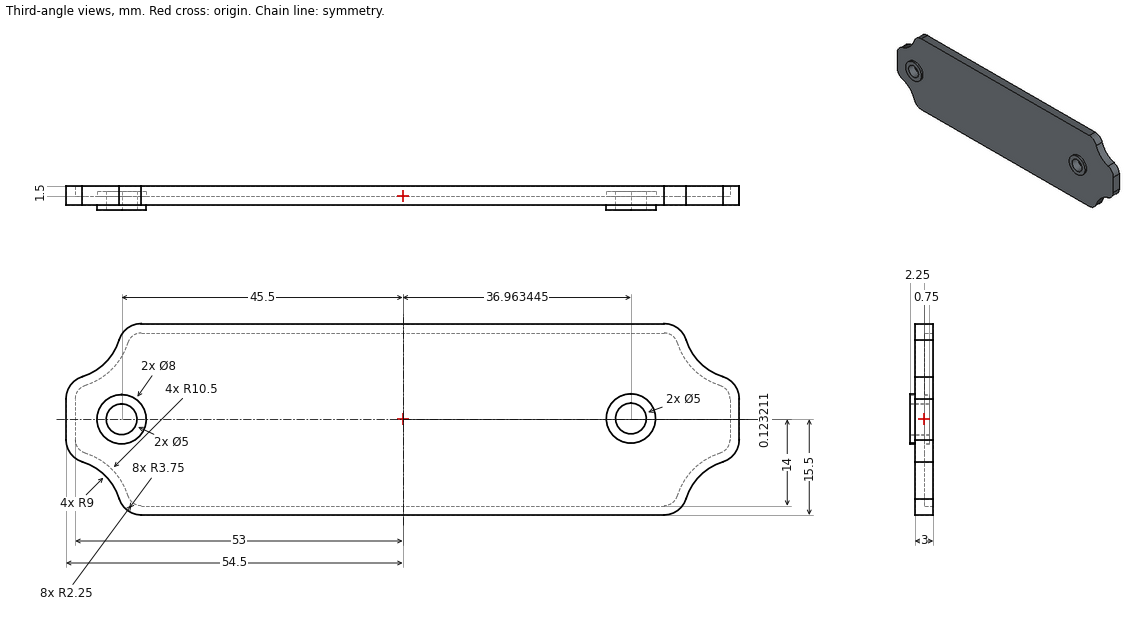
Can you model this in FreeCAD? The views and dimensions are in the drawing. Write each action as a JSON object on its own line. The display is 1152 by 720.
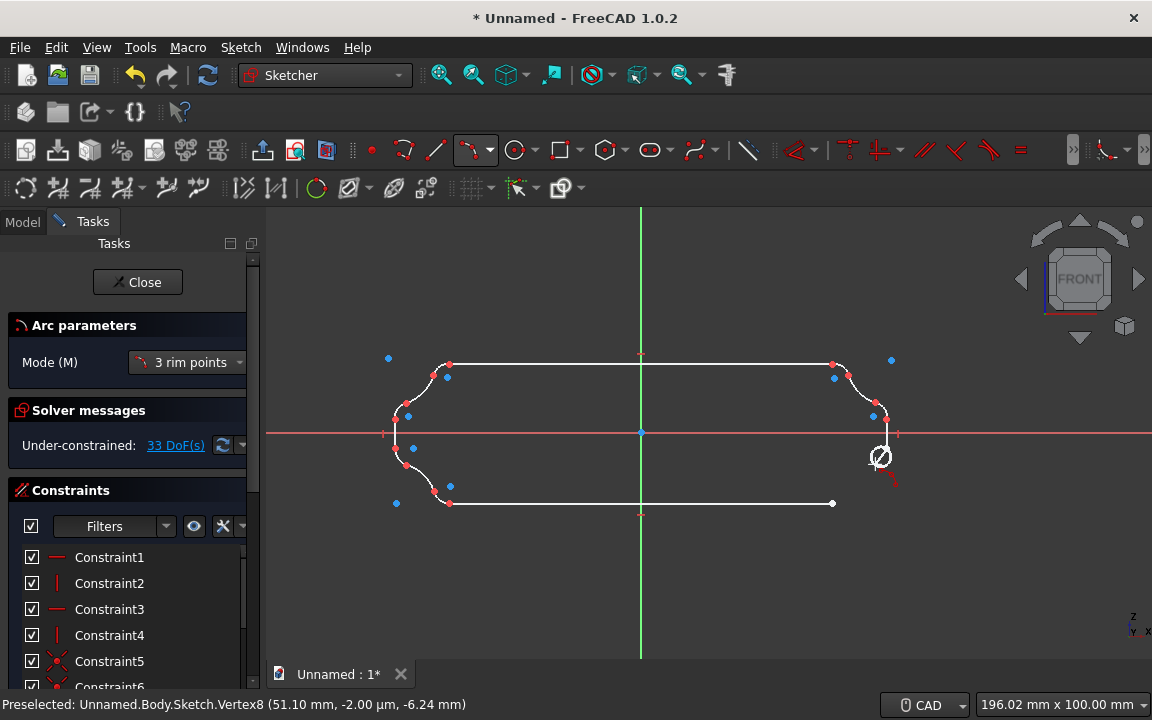
{"action": "scroll", "coordinate": [884, 458], "scroll_direction": "up", "scroll_amount": 8}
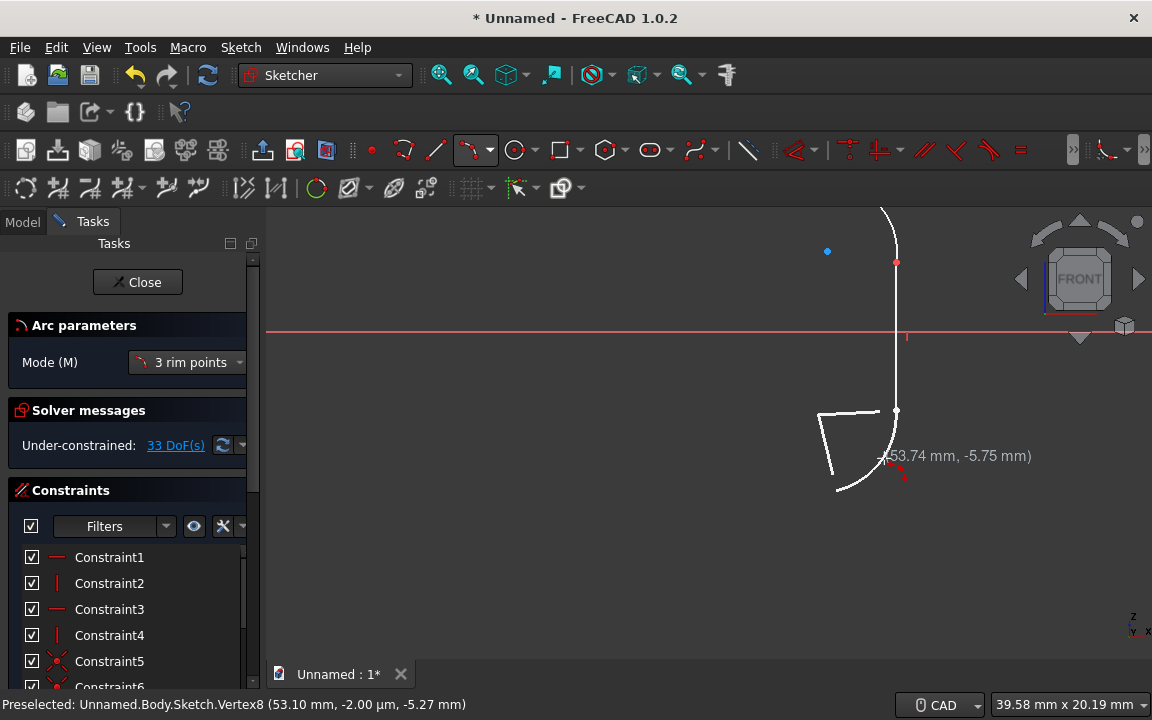
{"action": "left_click", "coordinate": [882, 456]}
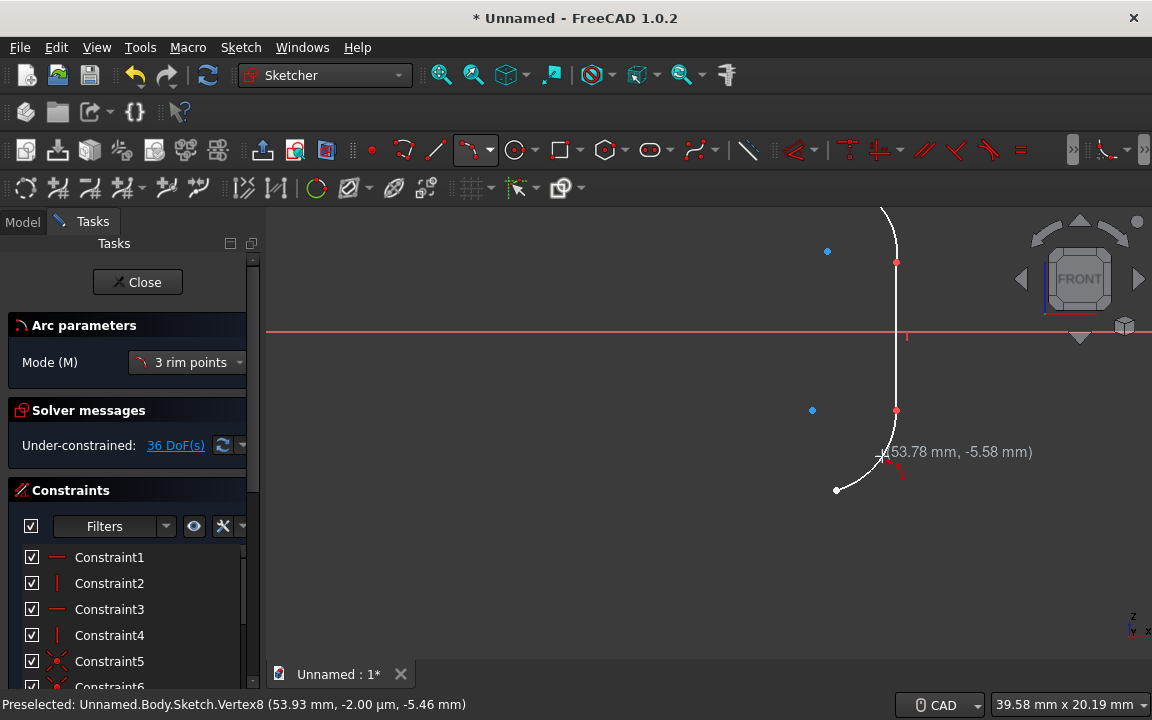
{"action": "scroll", "coordinate": [884, 459], "scroll_direction": "down", "scroll_amount": 8}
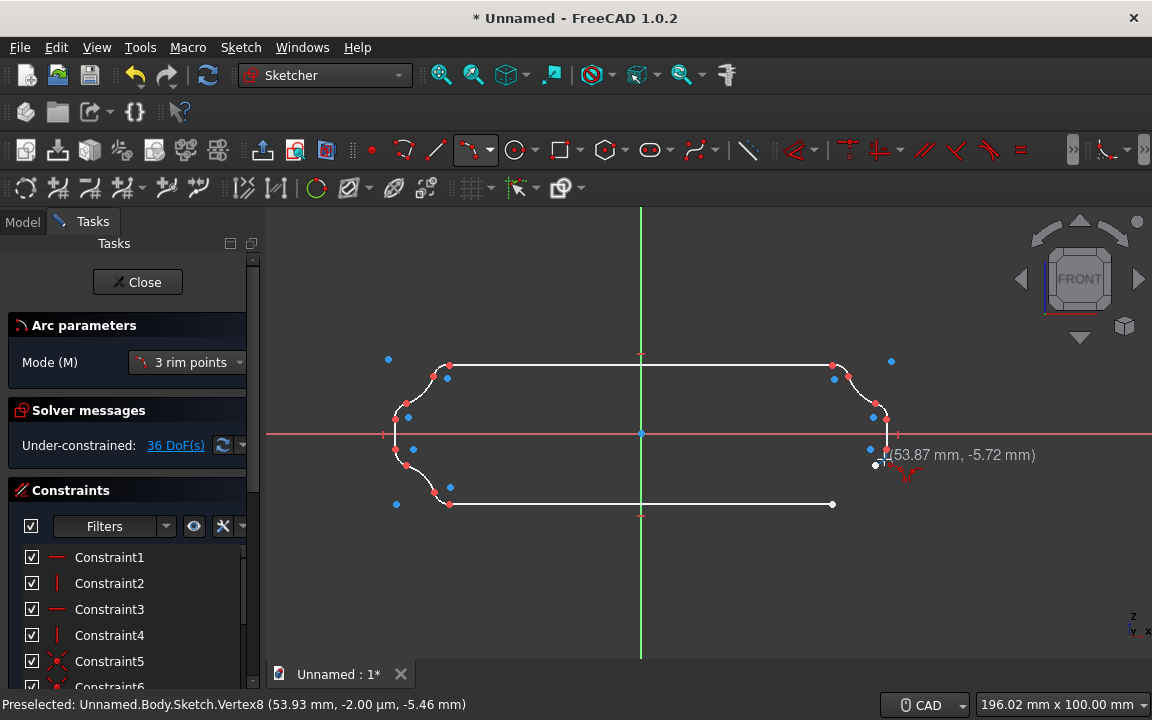
{"action": "left_click", "coordinate": [875, 466]}
{"action": "left_click", "coordinate": [849, 492]}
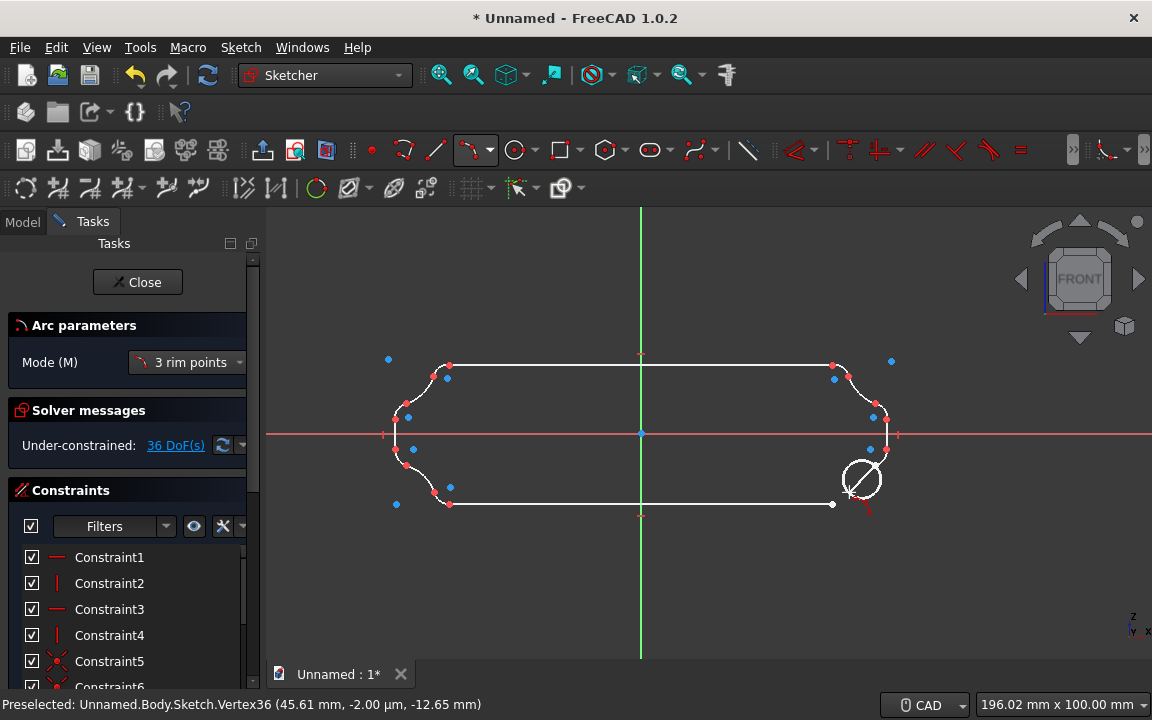
{"action": "scroll", "coordinate": [859, 475], "scroll_direction": "up", "scroll_amount": 7}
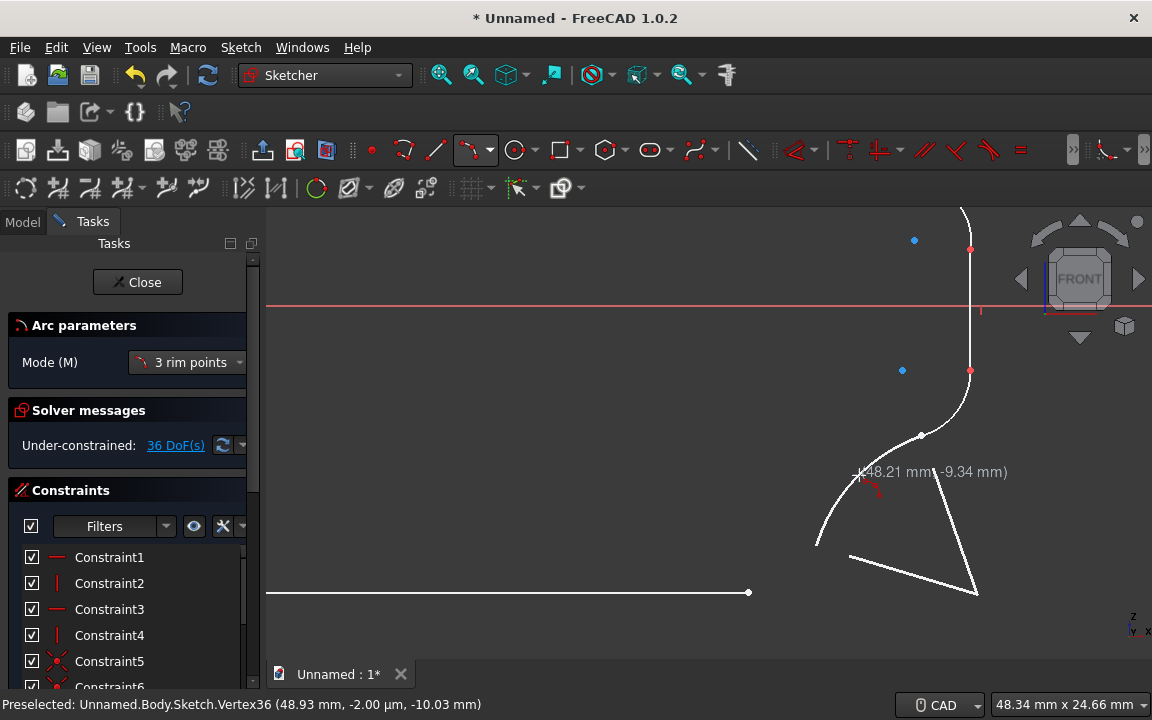
{"action": "left_click", "coordinate": [856, 474]}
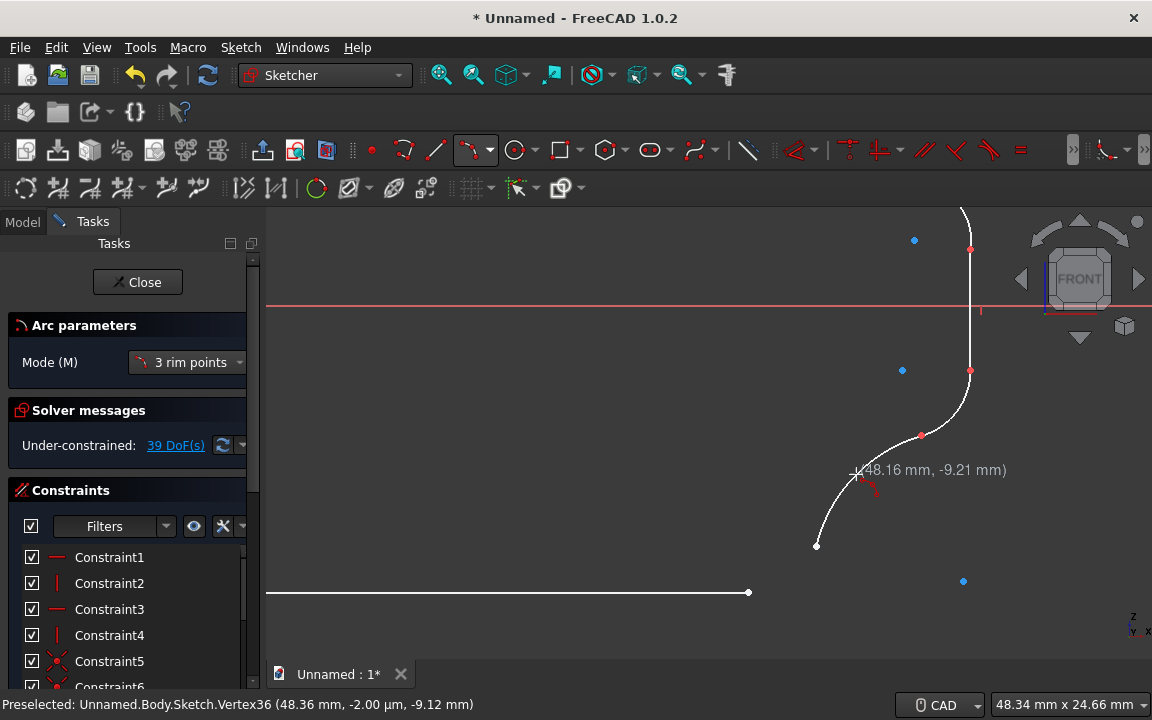
{"action": "scroll", "coordinate": [859, 475], "scroll_direction": "down", "scroll_amount": 7}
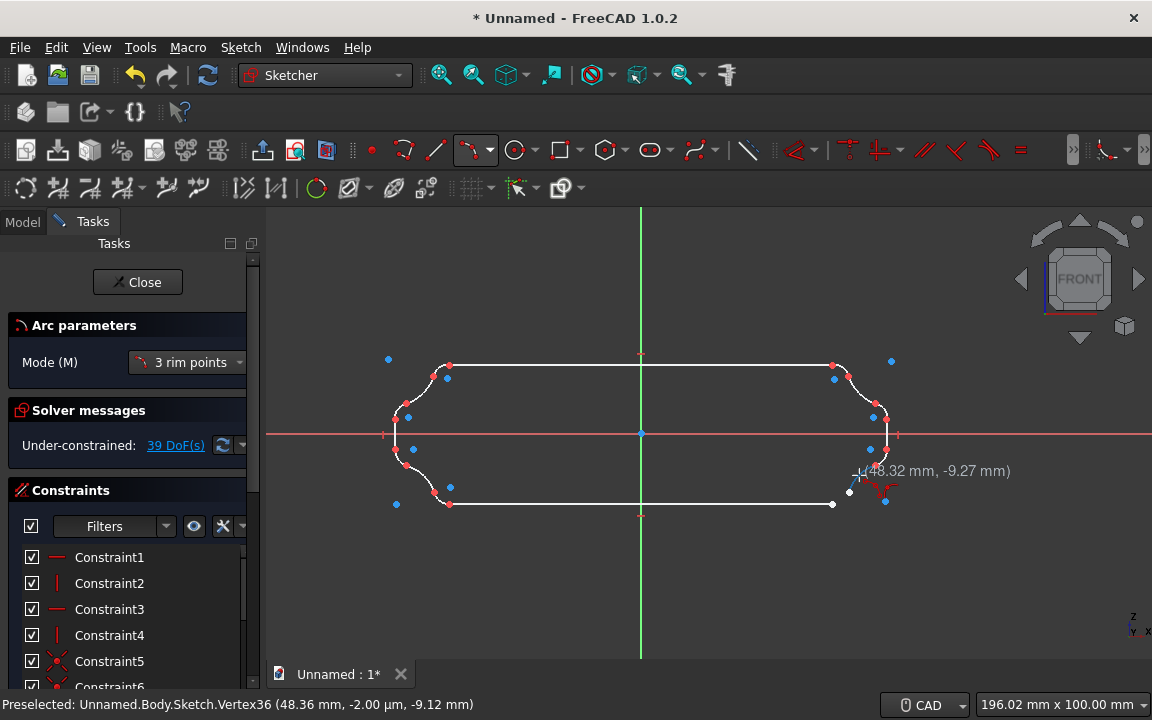
{"action": "left_click", "coordinate": [849, 493]}
{"action": "left_click", "coordinate": [832, 504]}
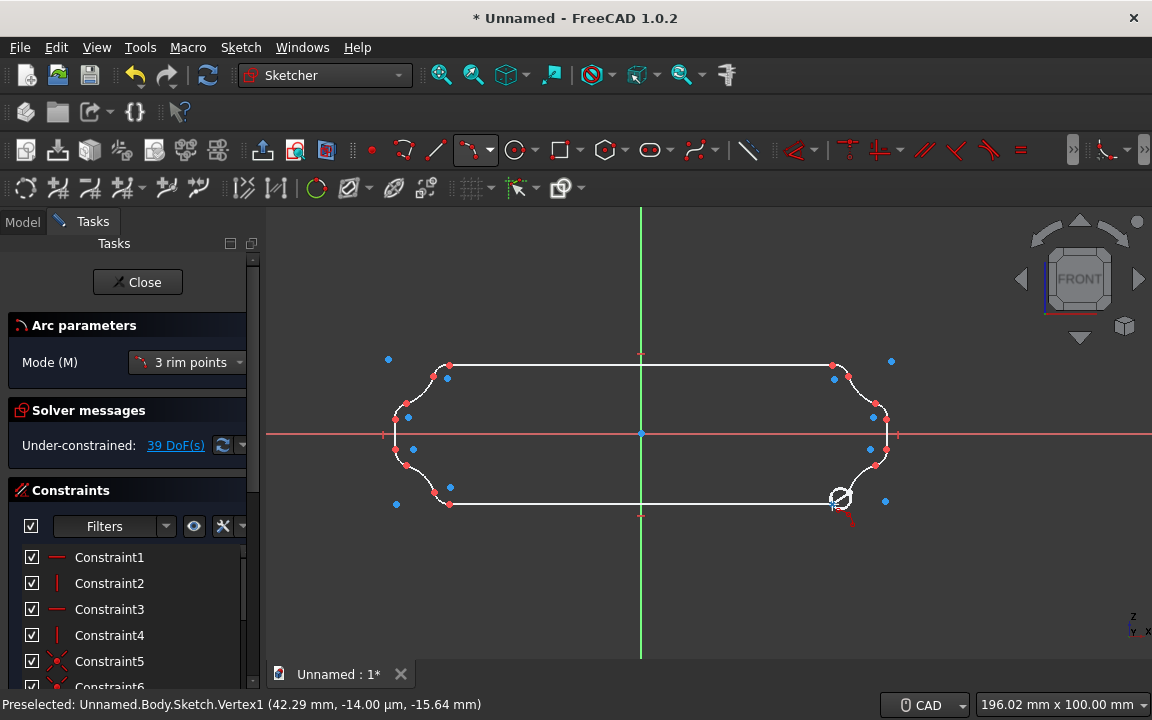
{"action": "scroll", "coordinate": [842, 501], "scroll_direction": "up", "scroll_amount": 8}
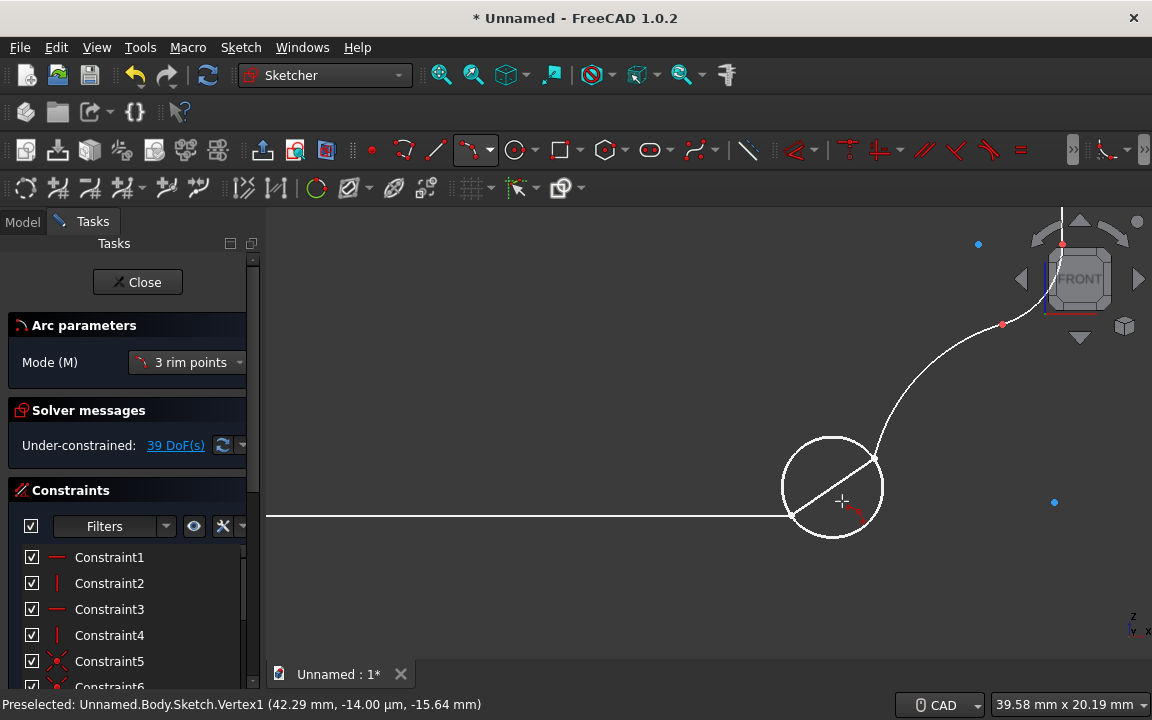
{"action": "left_click", "coordinate": [841, 496]}
{"action": "key", "text": "Escape"}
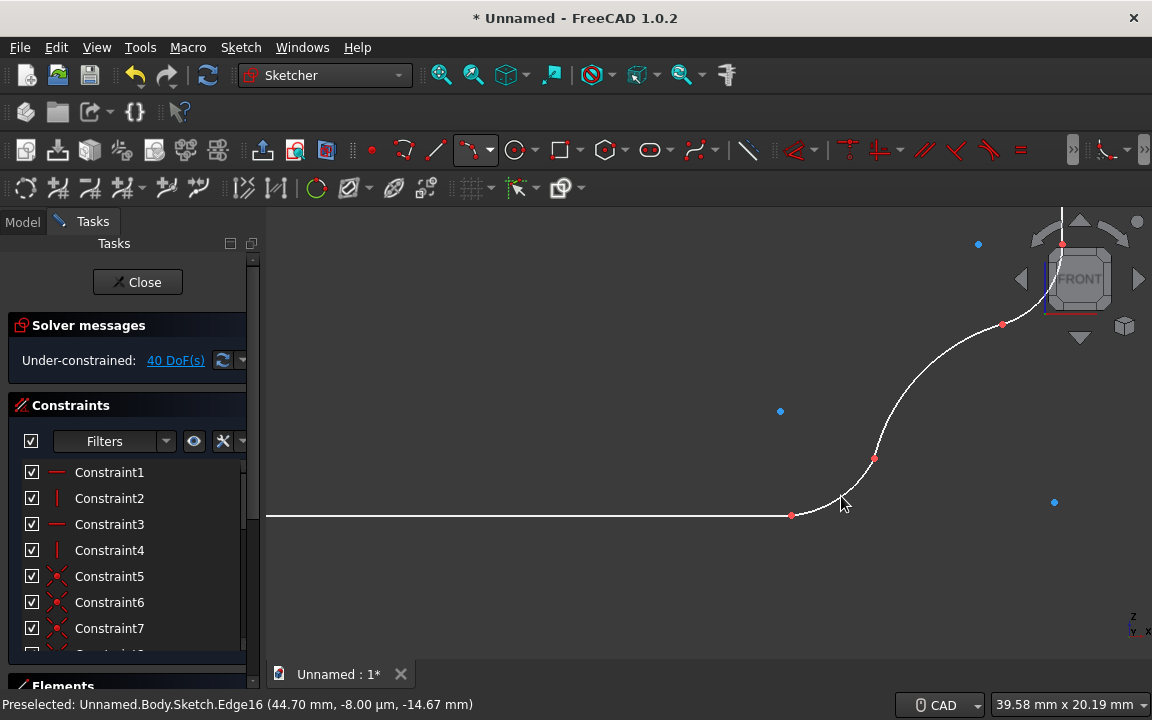
{"action": "scroll", "coordinate": [842, 501], "scroll_direction": "down", "scroll_amount": 8}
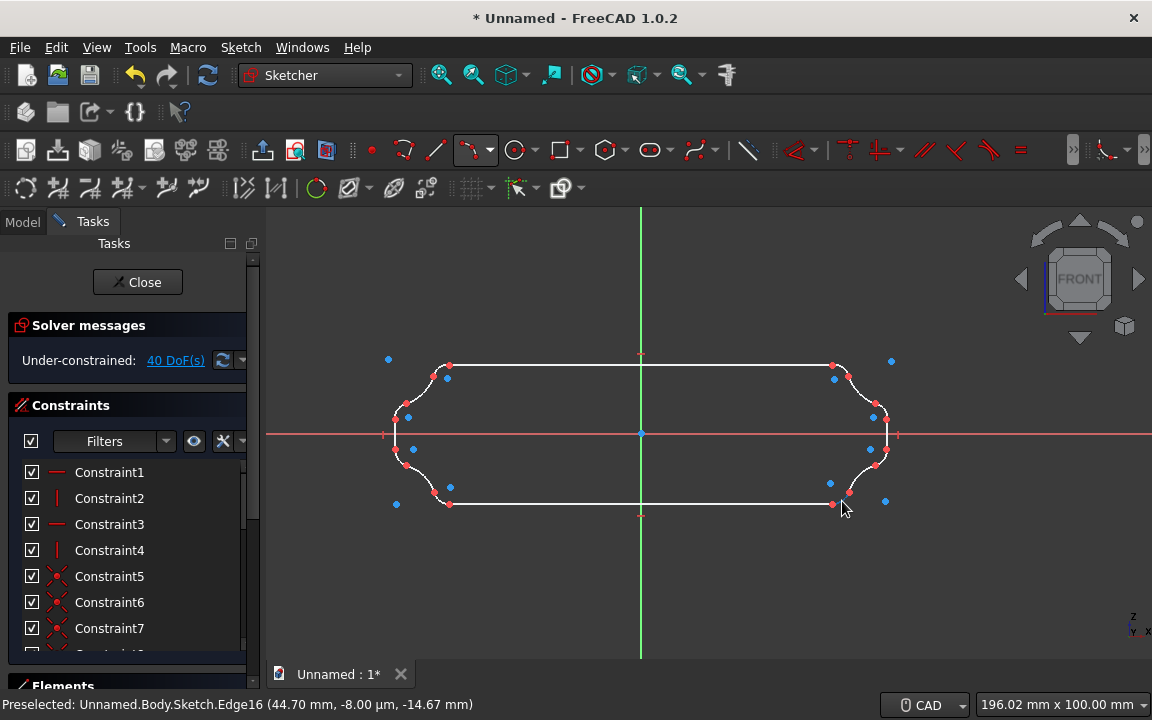
{"action": "left_click", "coordinate": [756, 504]}